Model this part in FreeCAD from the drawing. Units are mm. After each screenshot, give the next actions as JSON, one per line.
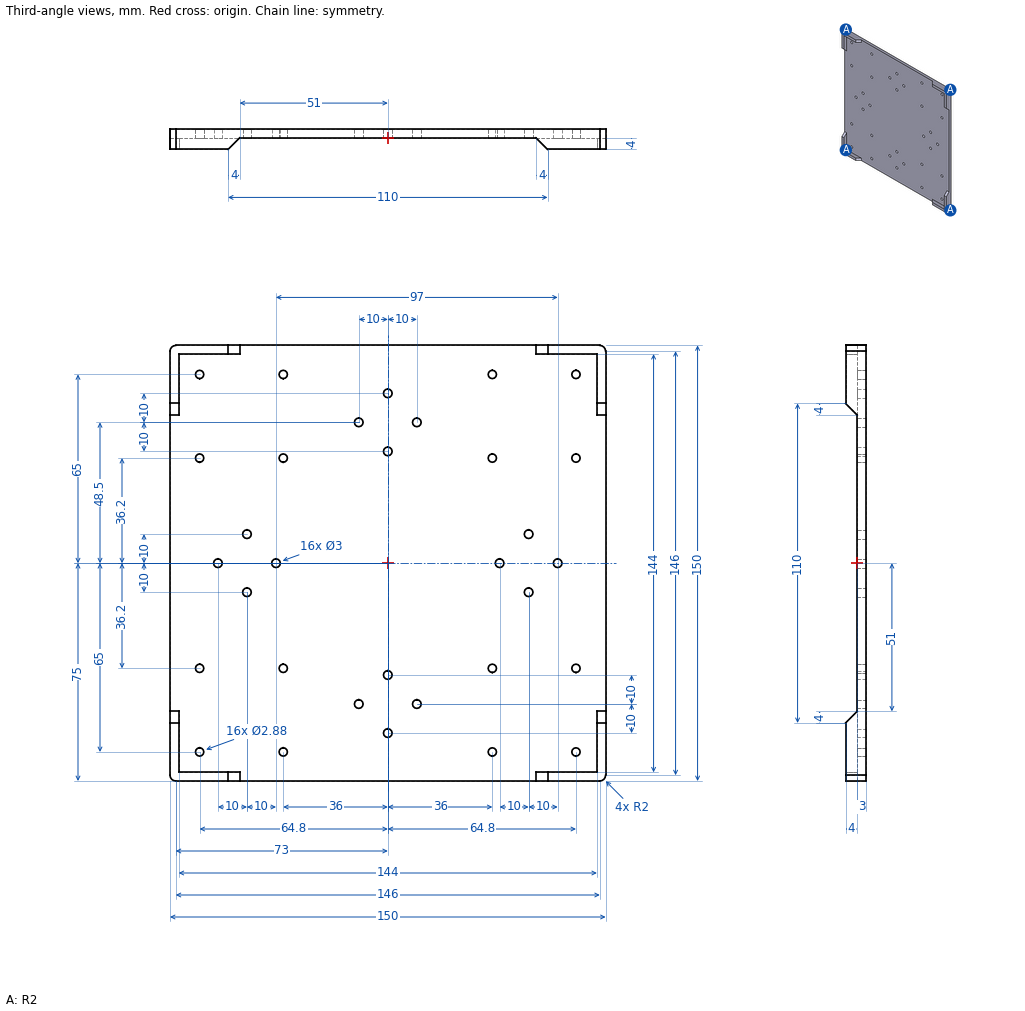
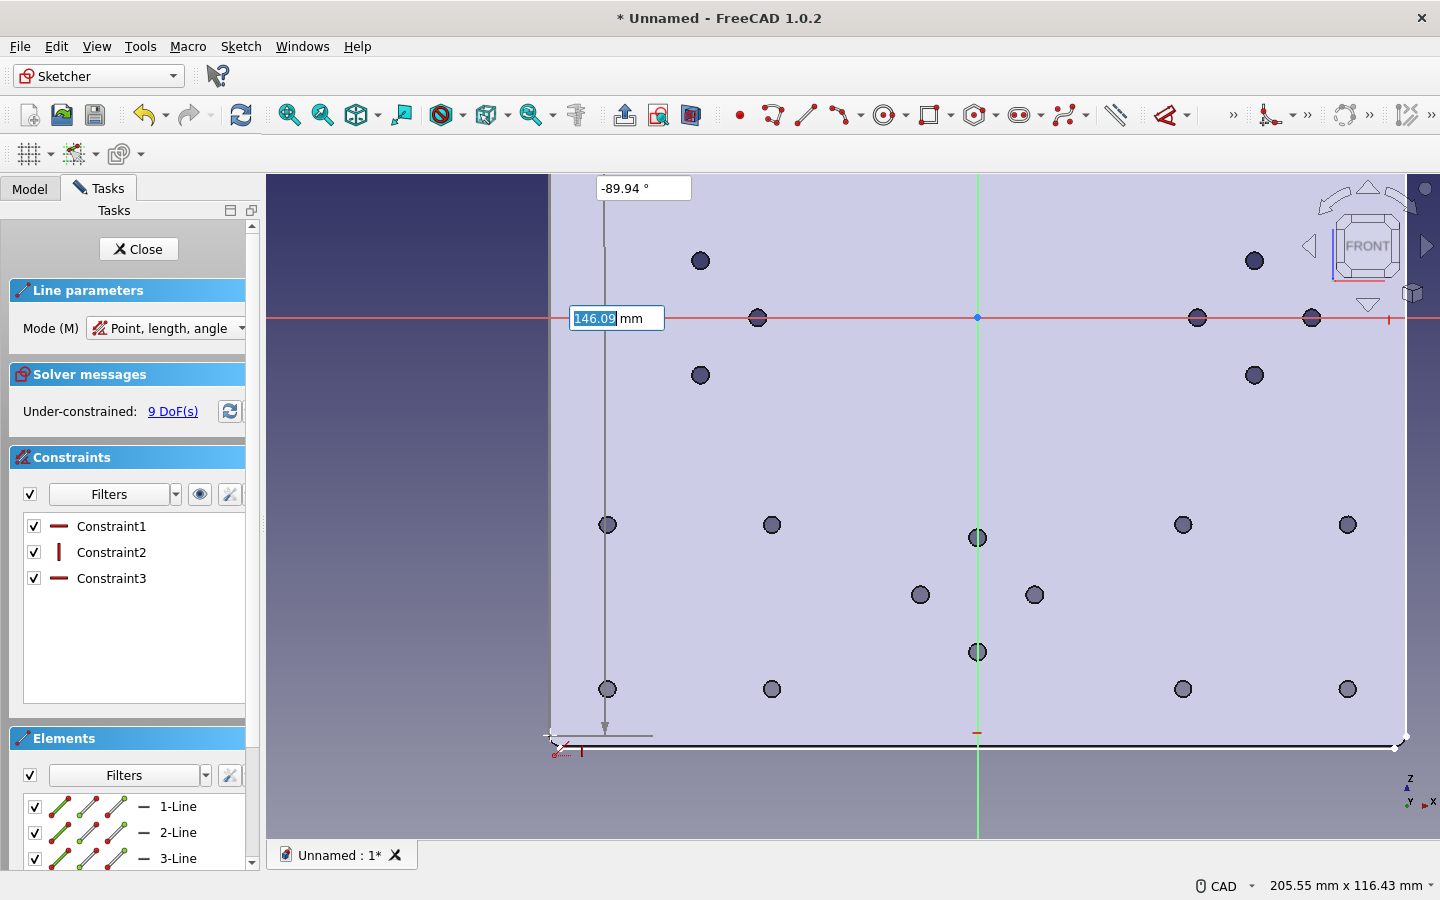
{"action": "left_click", "coordinate": [549, 735]}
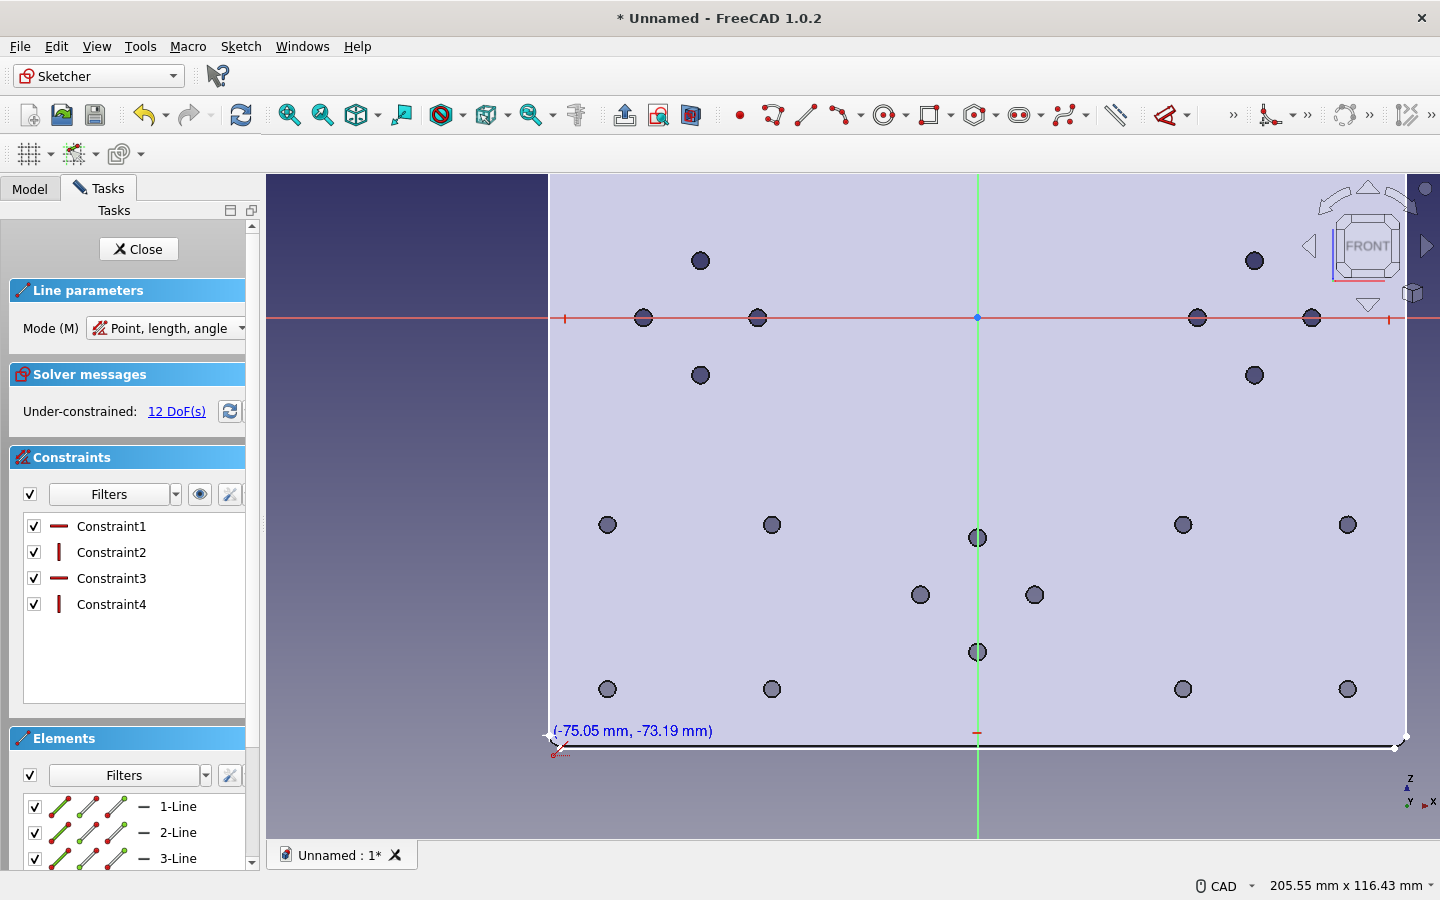
{"action": "key", "text": "g 3 a"}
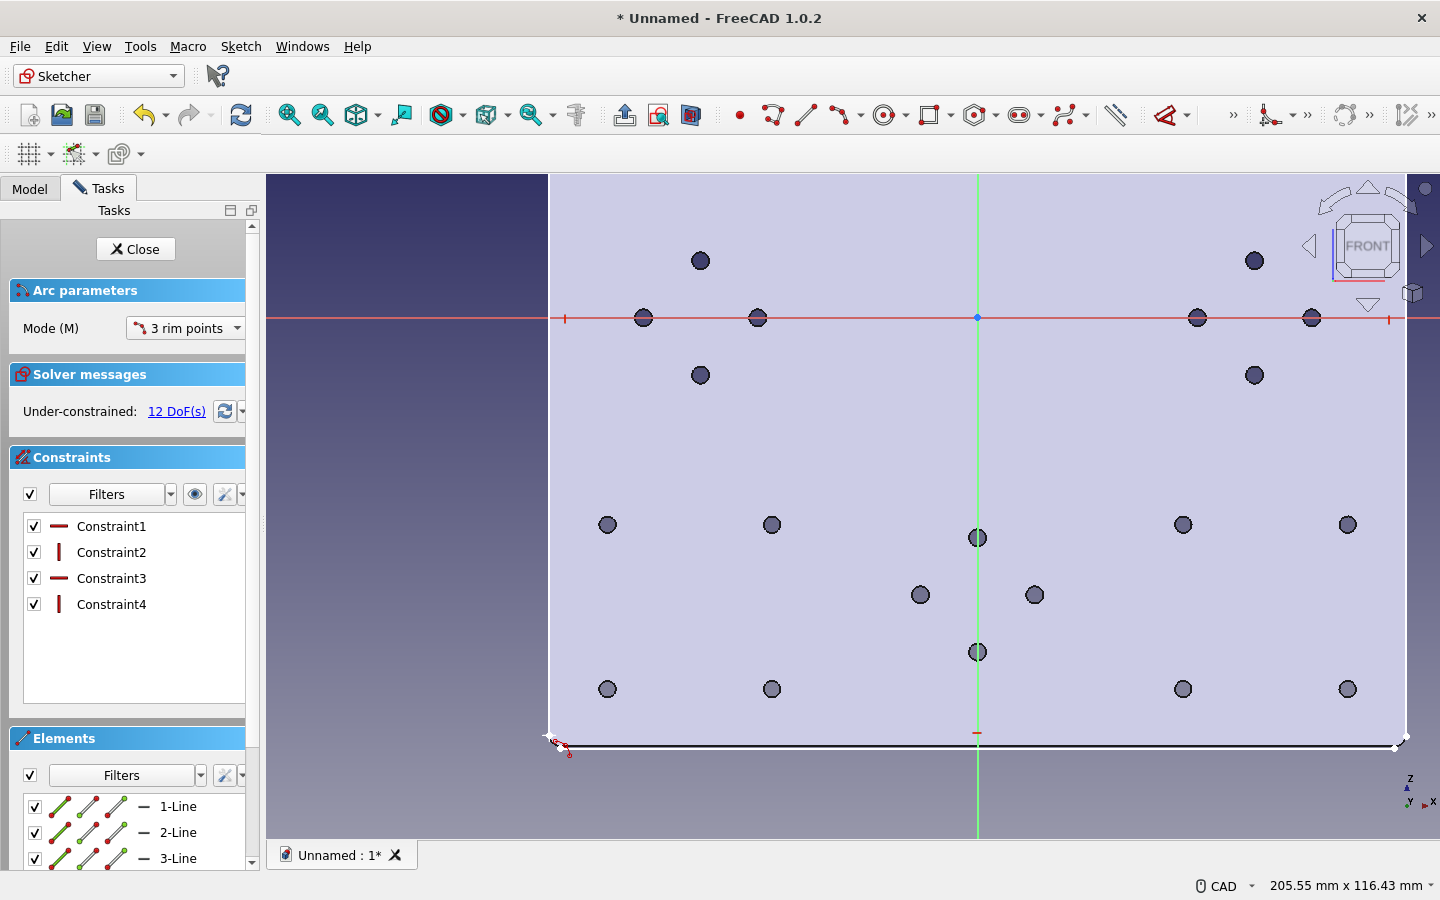
{"action": "scroll", "coordinate": [550, 736], "scroll_direction": "down", "scroll_amount": 3}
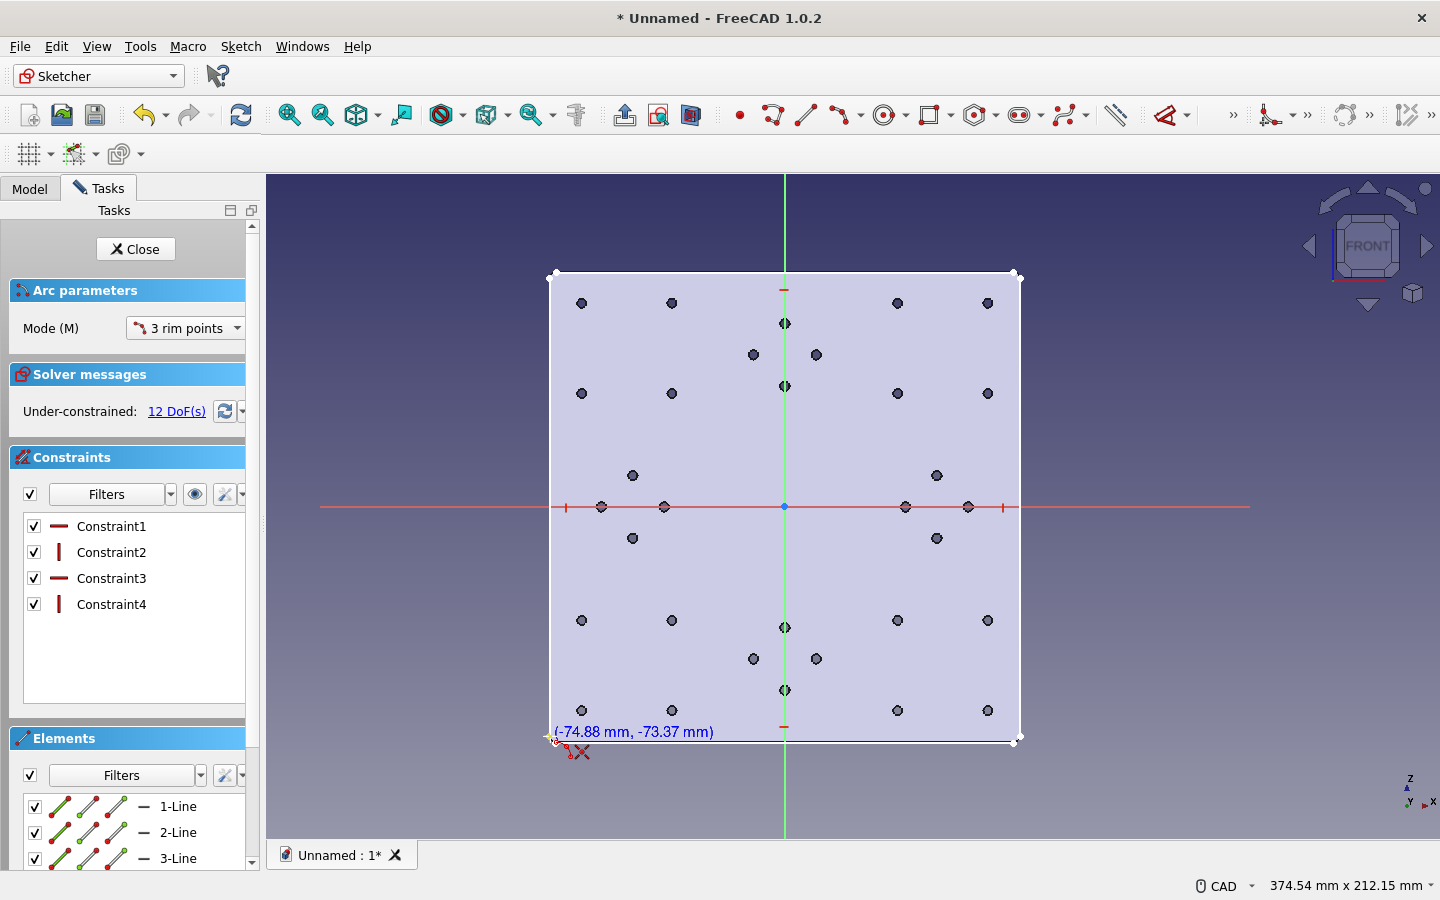
{"action": "scroll", "coordinate": [1014, 742], "scroll_direction": "up", "scroll_amount": 3}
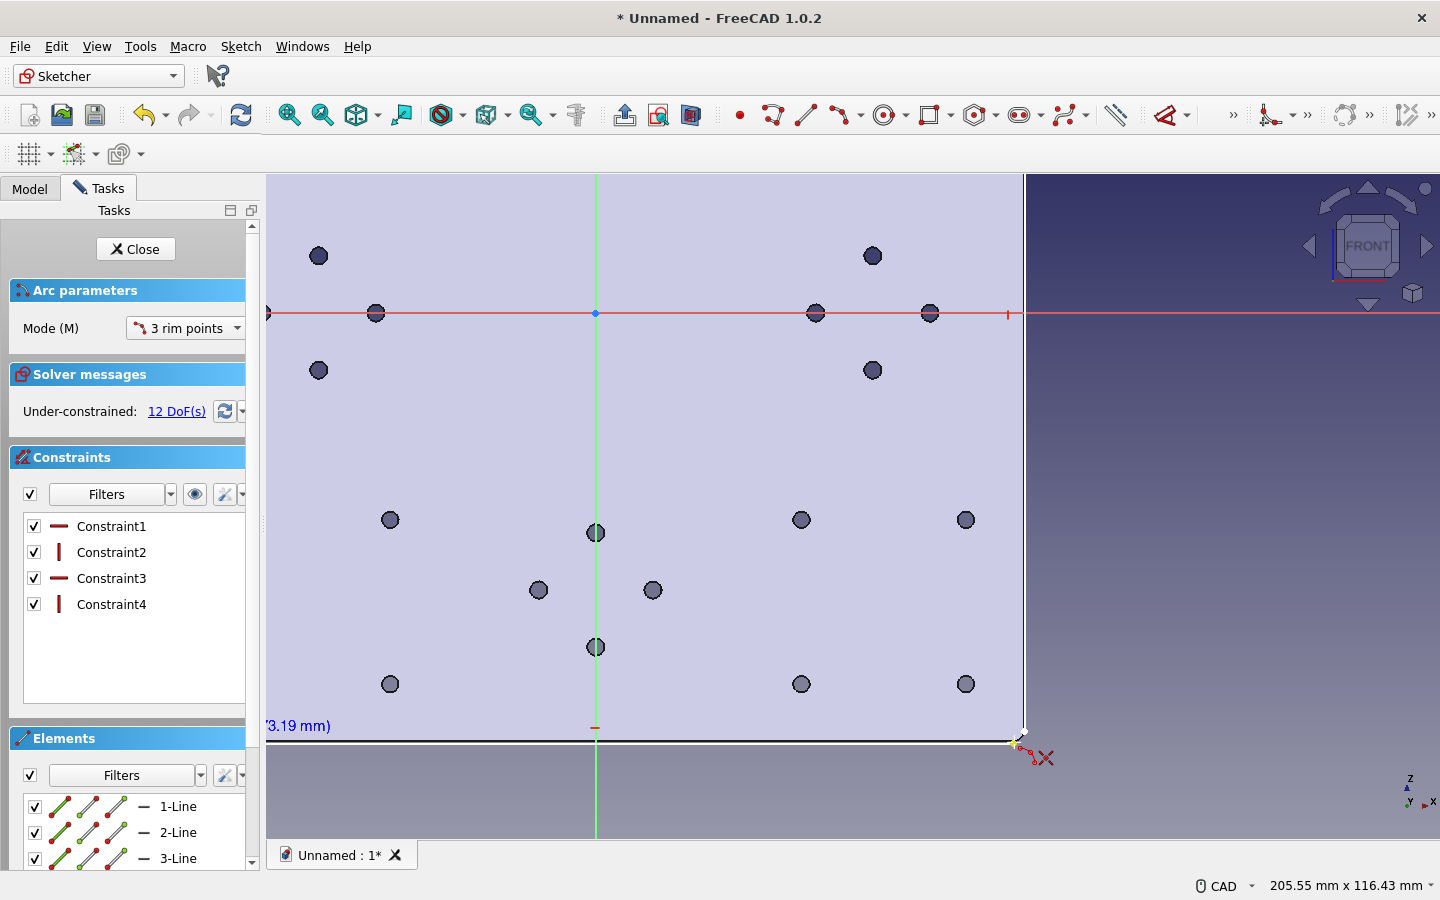
{"action": "left_click", "coordinate": [1013, 744]}
{"action": "left_click", "coordinate": [1025, 731]}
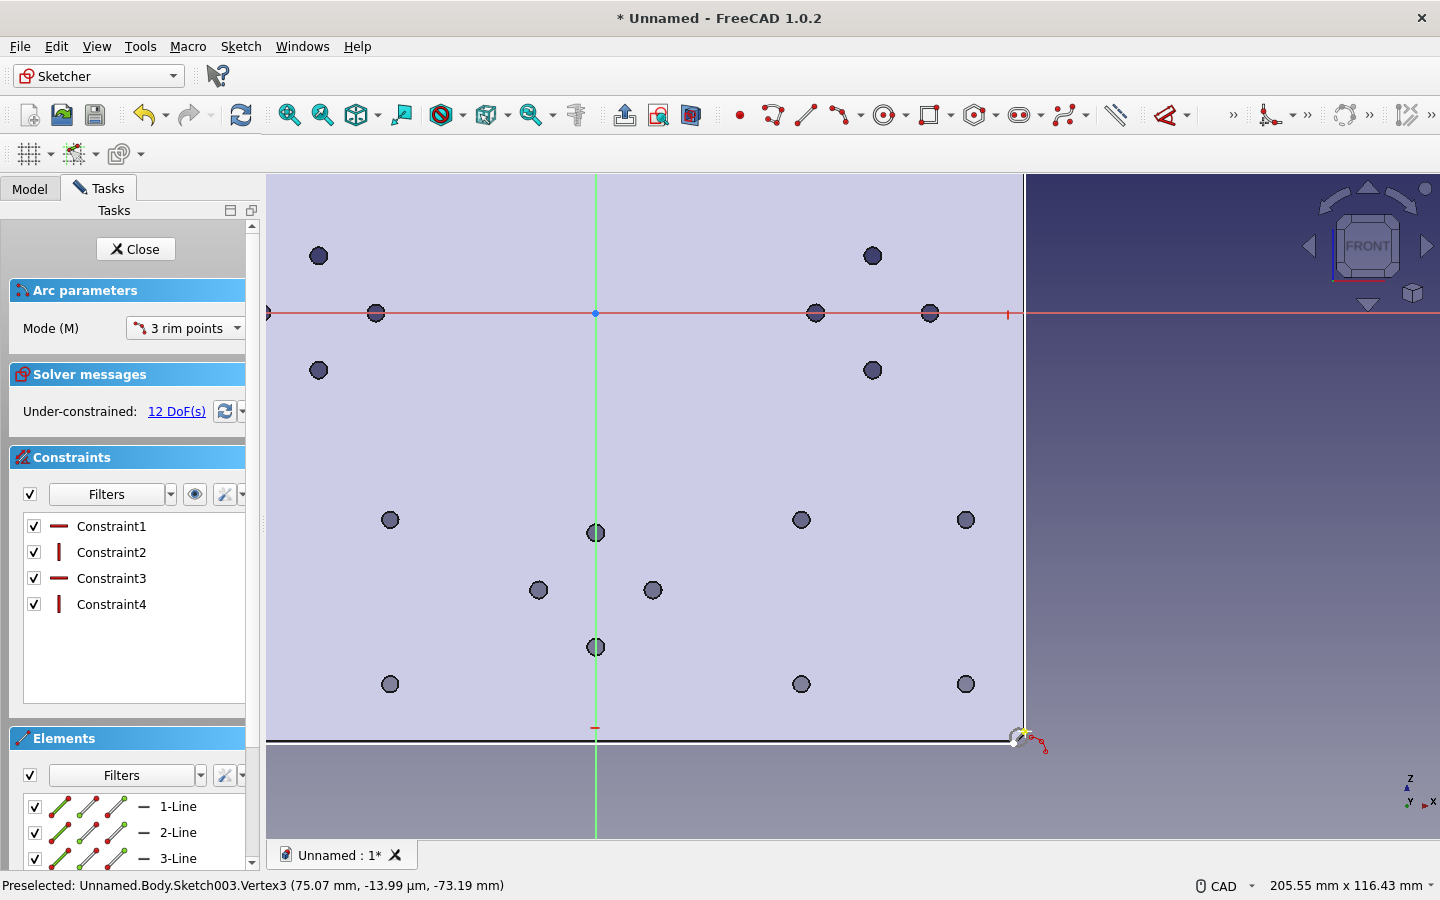
{"action": "scroll", "coordinate": [1021, 738], "scroll_direction": "up", "scroll_amount": 8}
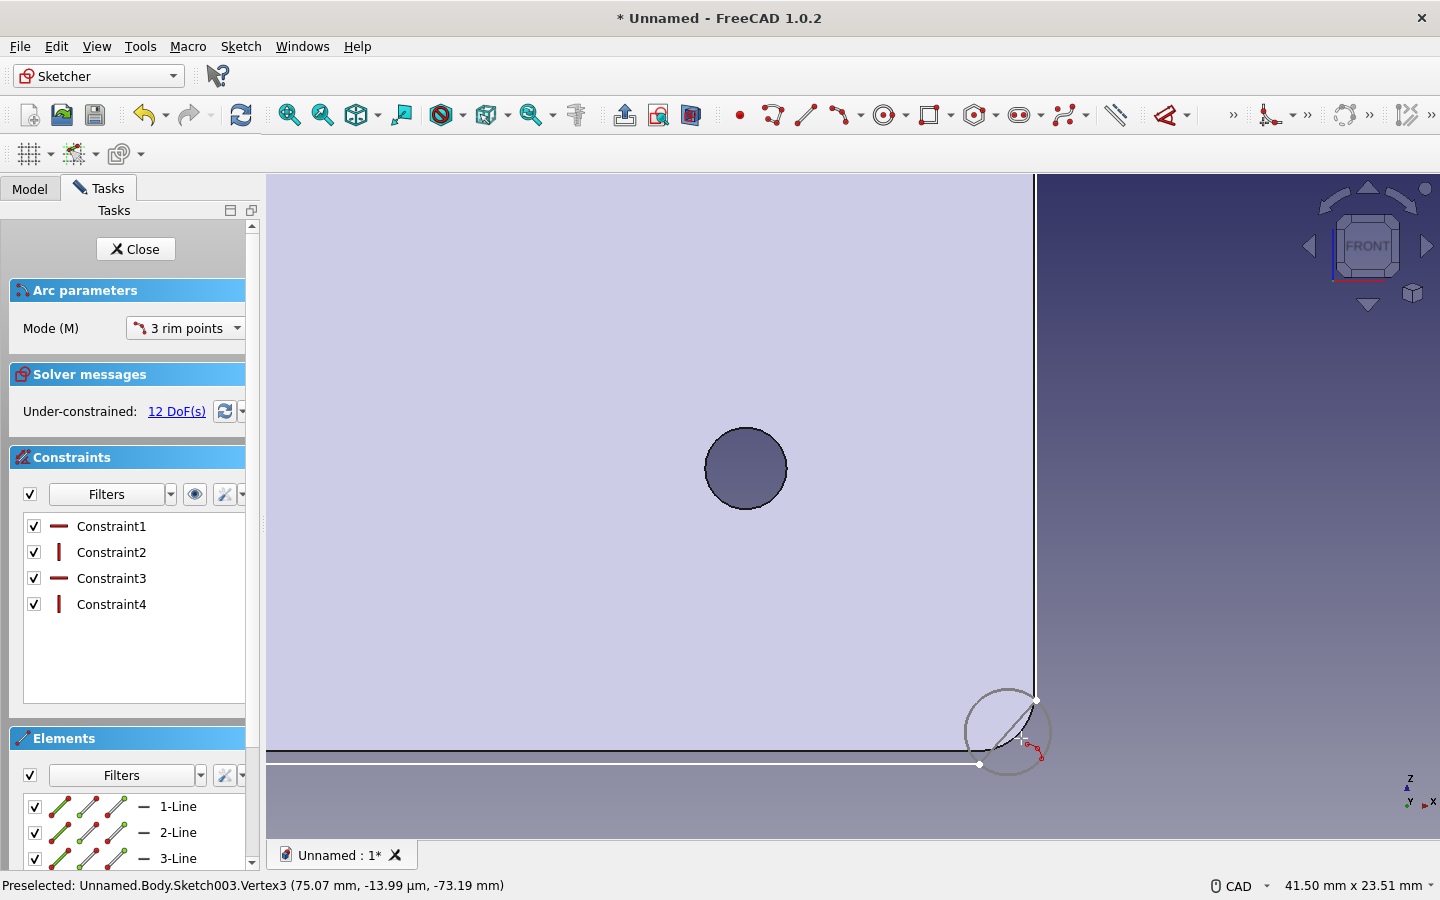
{"action": "left_click", "coordinate": [1018, 735]}